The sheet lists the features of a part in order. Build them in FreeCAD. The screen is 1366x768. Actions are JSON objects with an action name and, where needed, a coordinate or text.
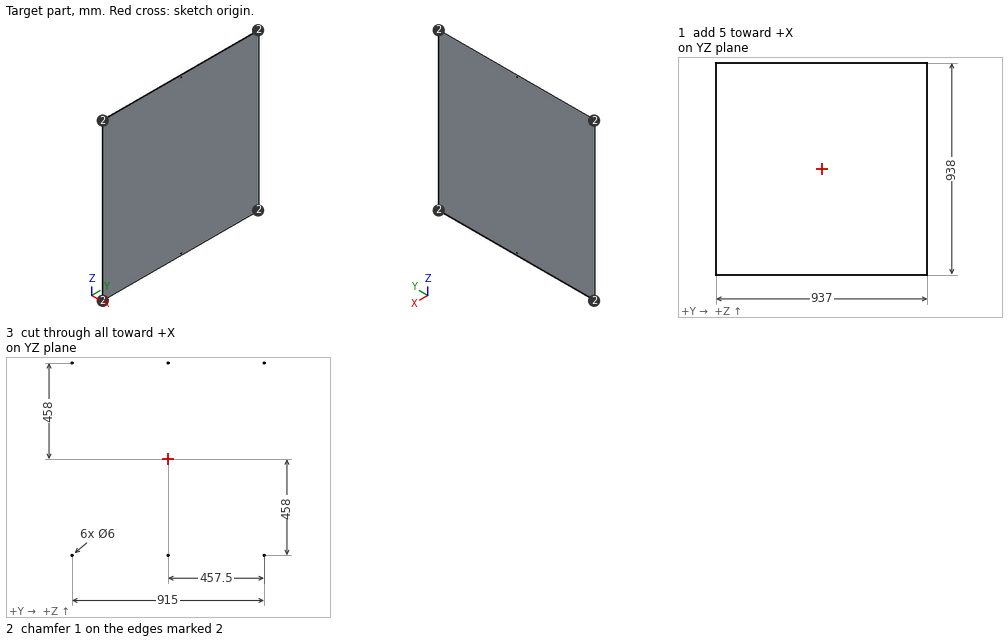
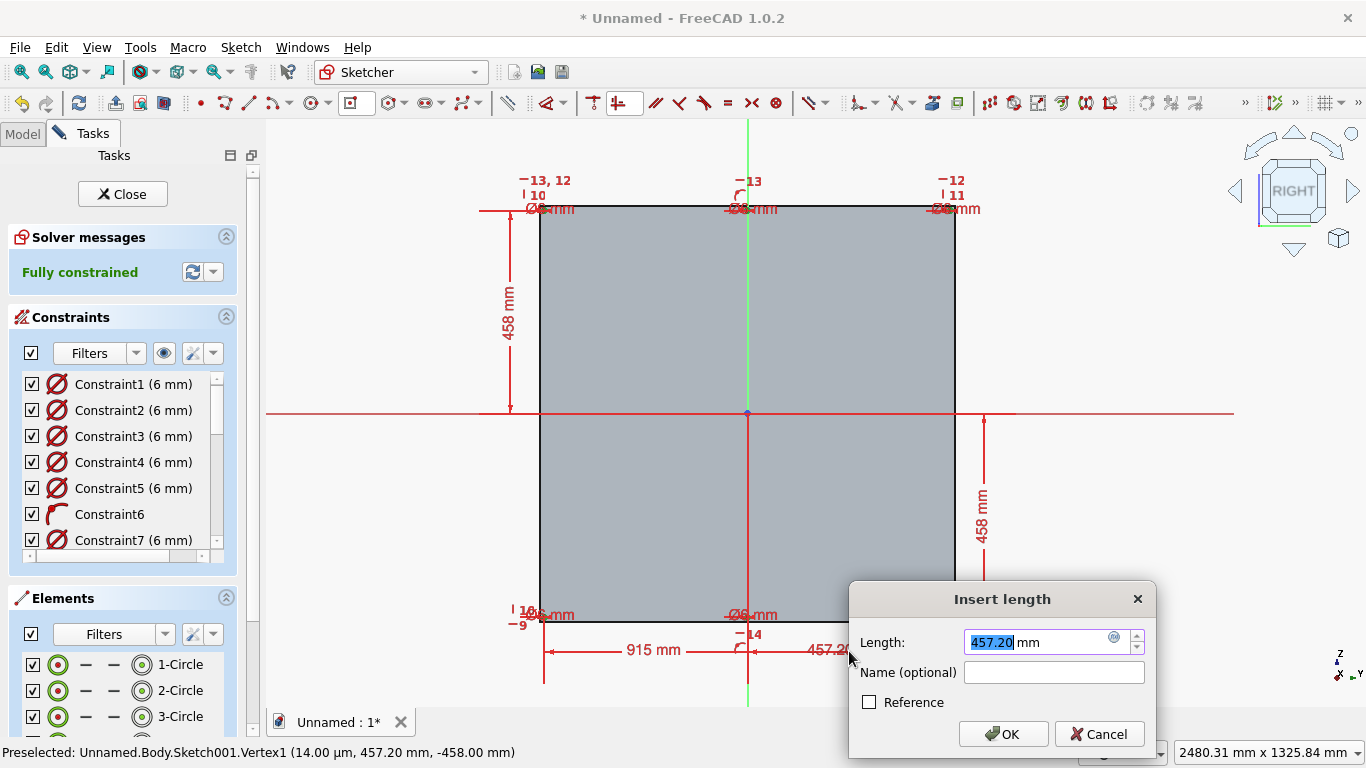
{"action": "type", "text": "457.5"}
{"action": "key", "text": "Return"}
{"action": "key", "text": "Escape"}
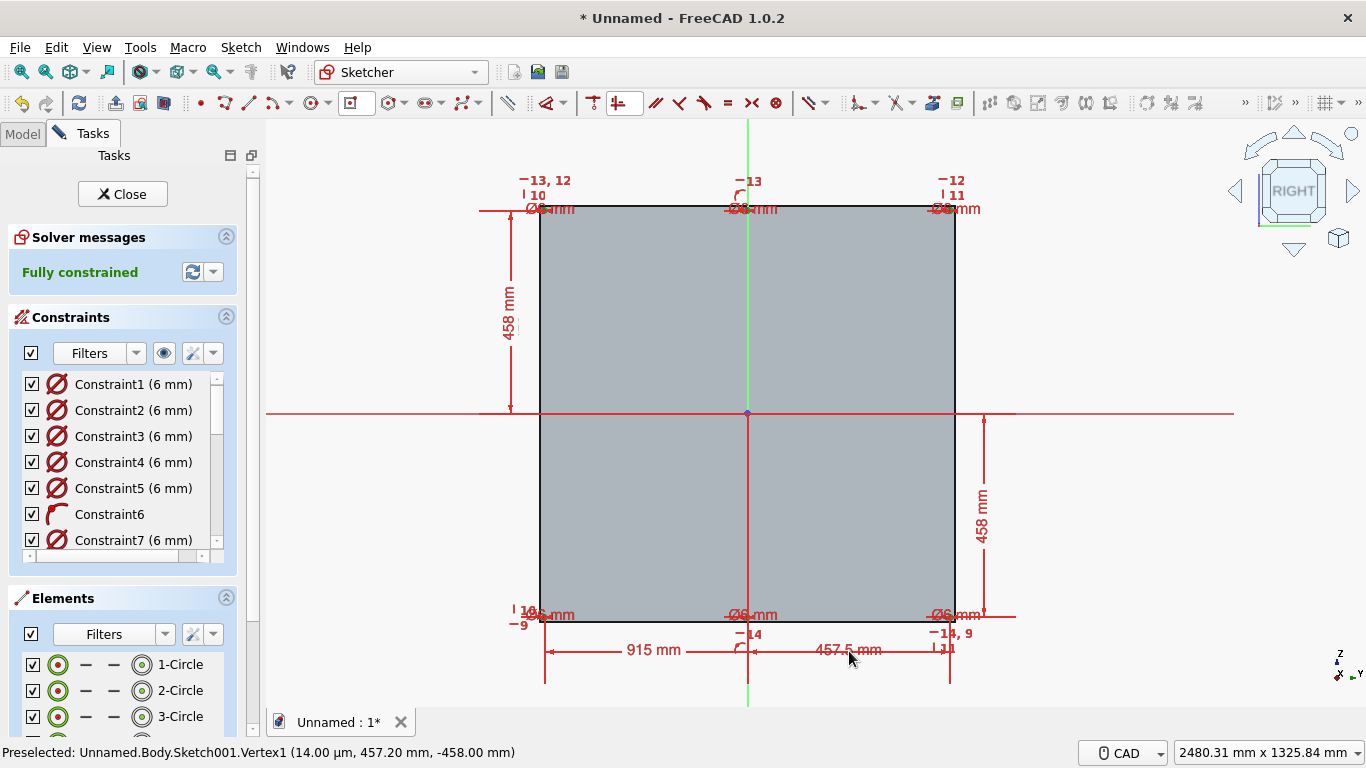
{"action": "left_click", "coordinate": [123, 194]}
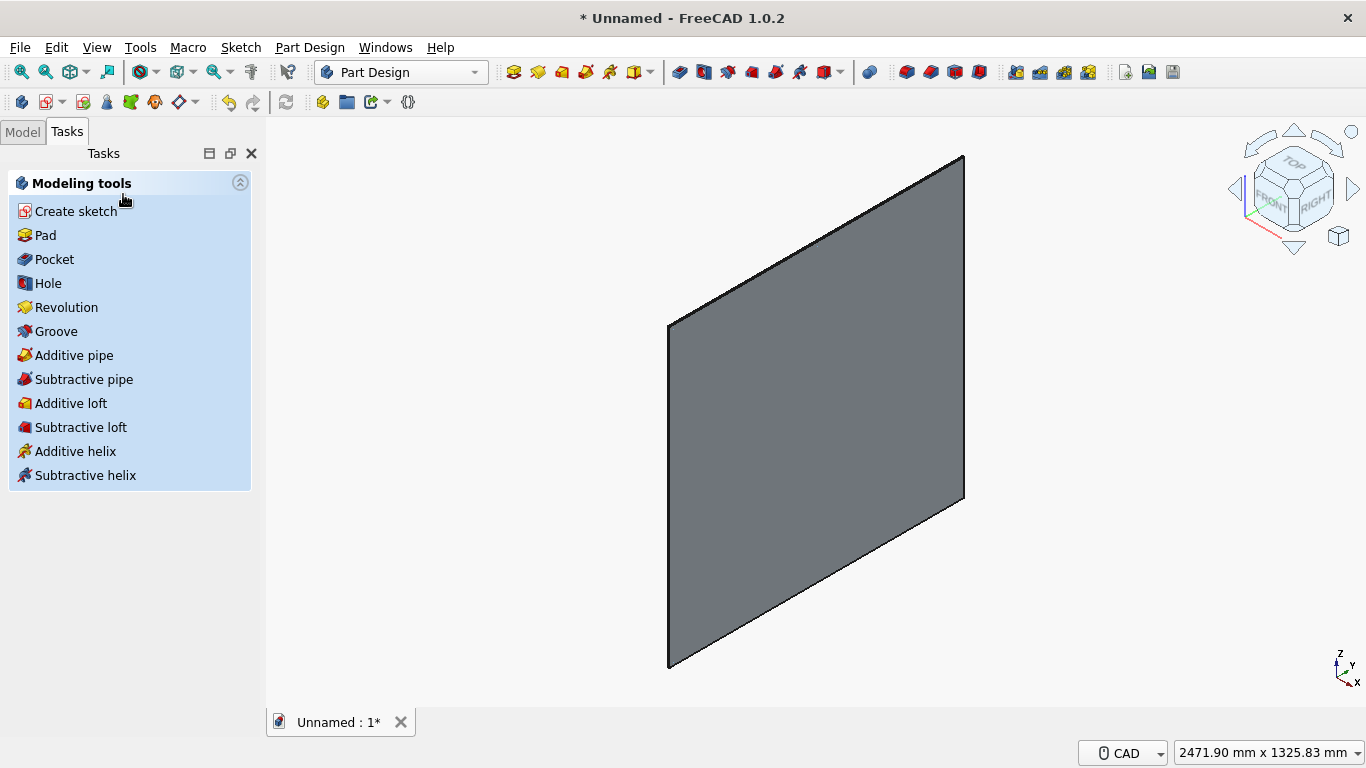
{"action": "left_click", "coordinate": [680, 72]}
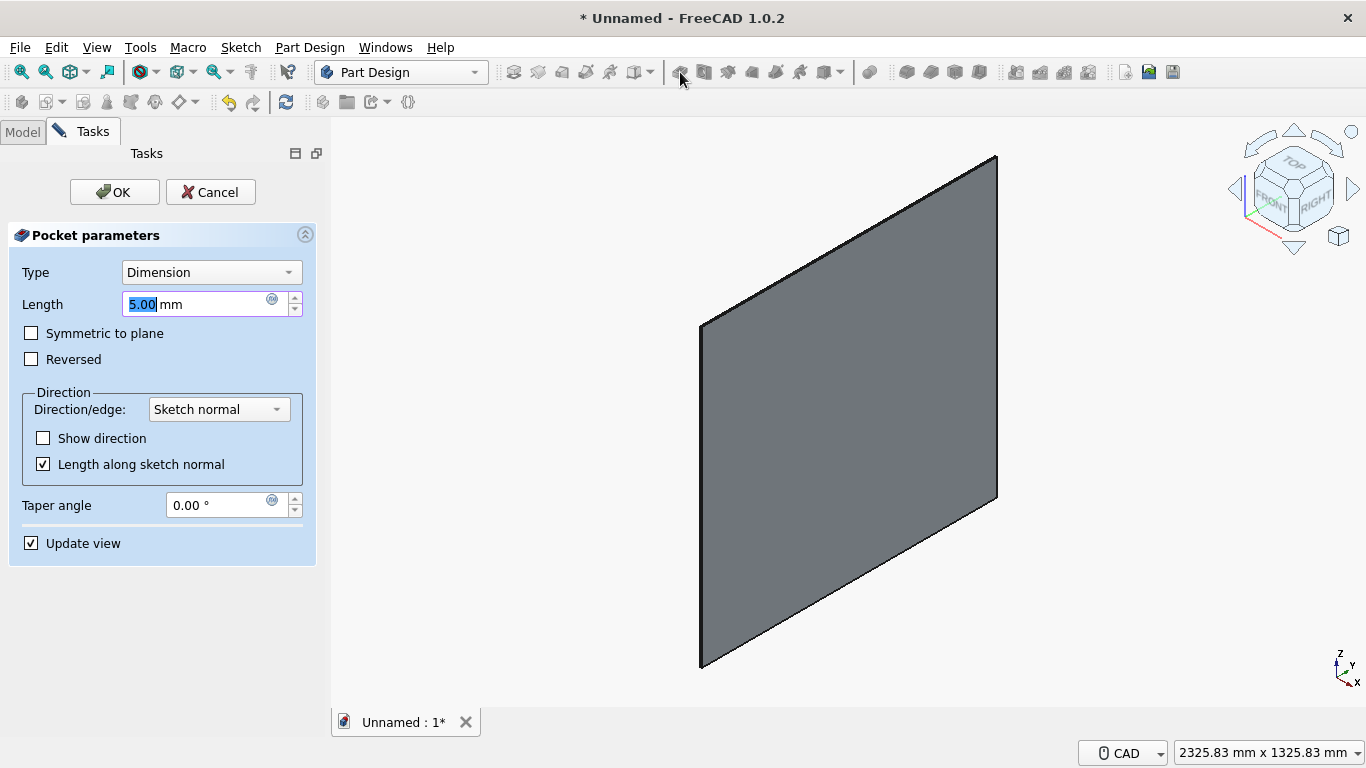
{"action": "left_click", "coordinate": [212, 272]}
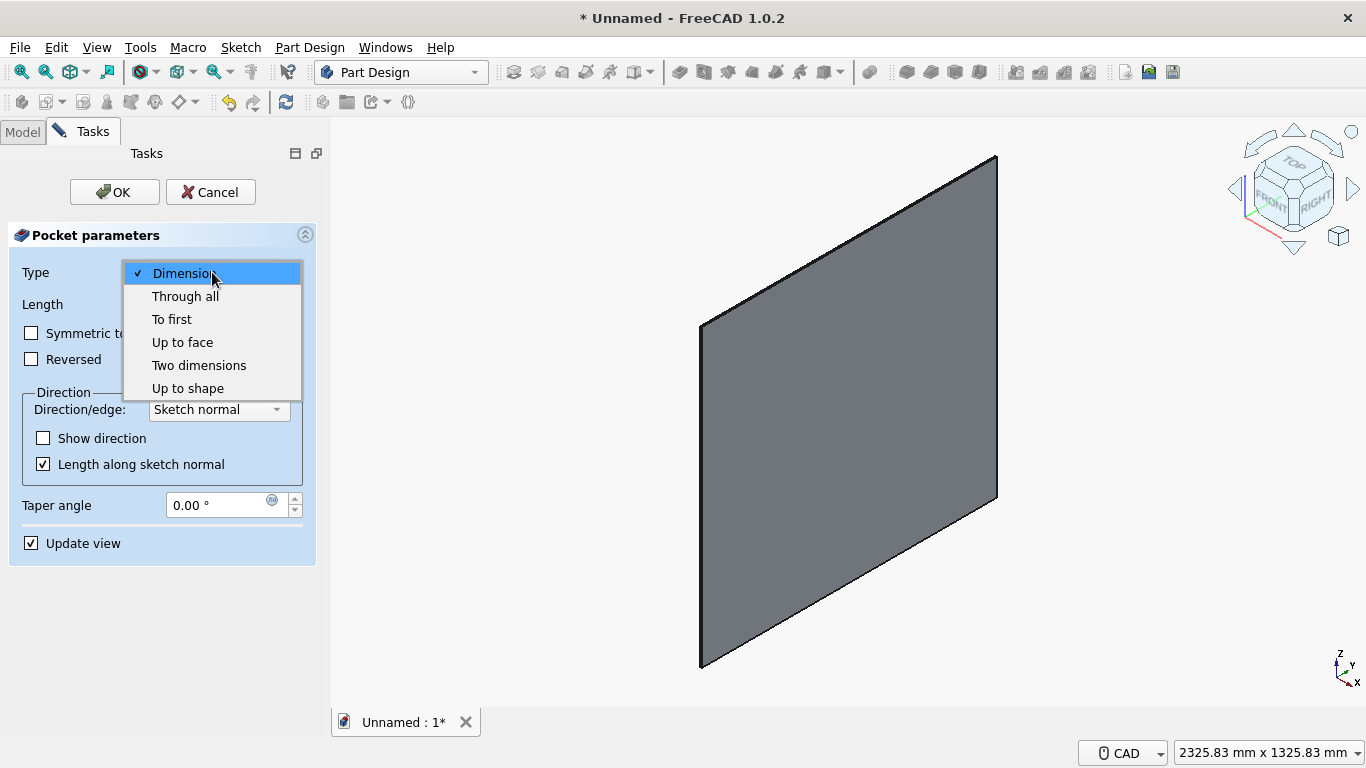
{"action": "left_click", "coordinate": [212, 296]}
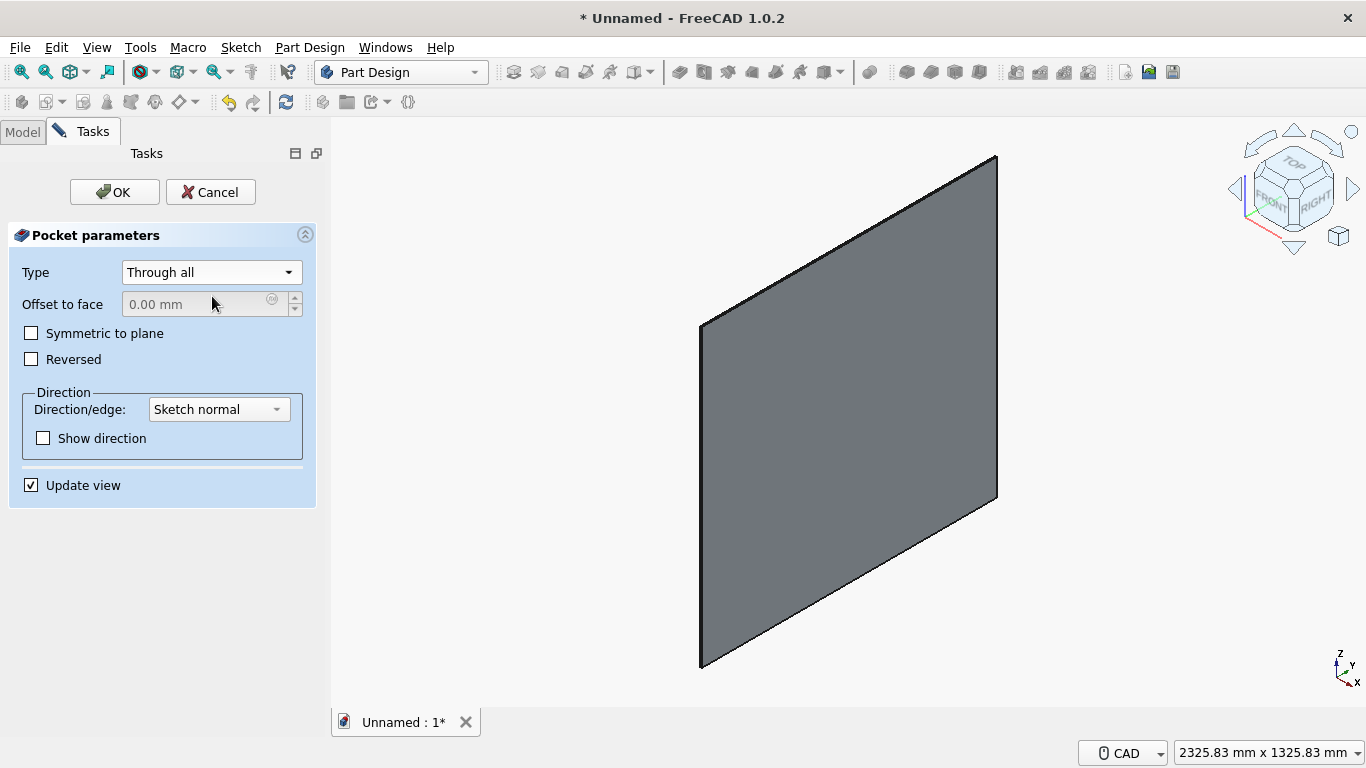
{"action": "left_click", "coordinate": [30, 359]}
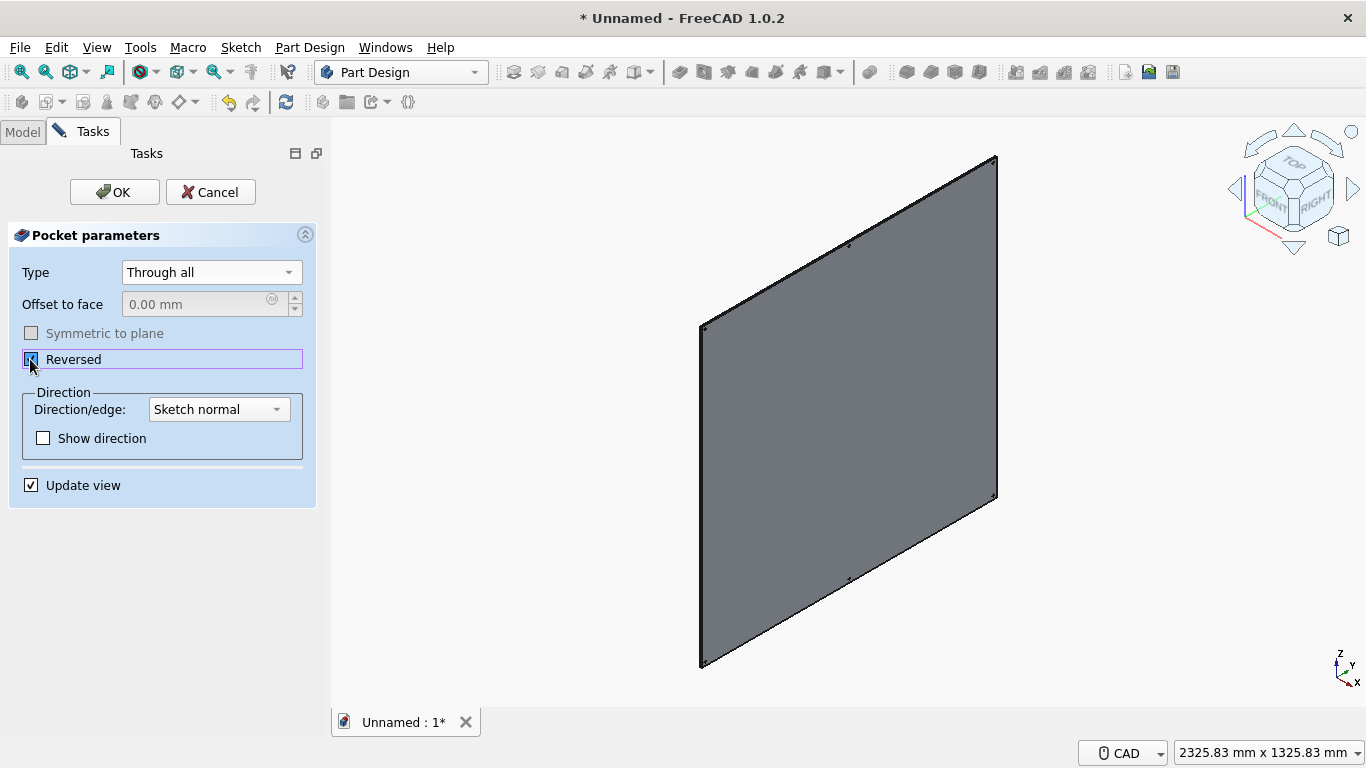
{"action": "left_click", "coordinate": [115, 192]}